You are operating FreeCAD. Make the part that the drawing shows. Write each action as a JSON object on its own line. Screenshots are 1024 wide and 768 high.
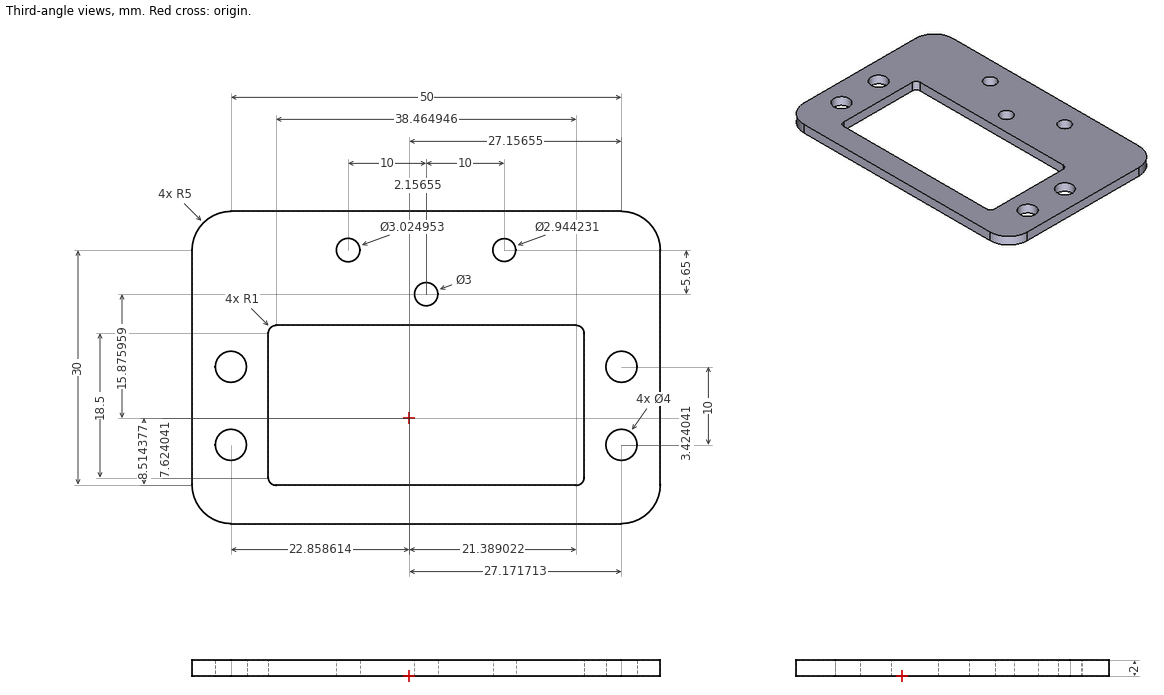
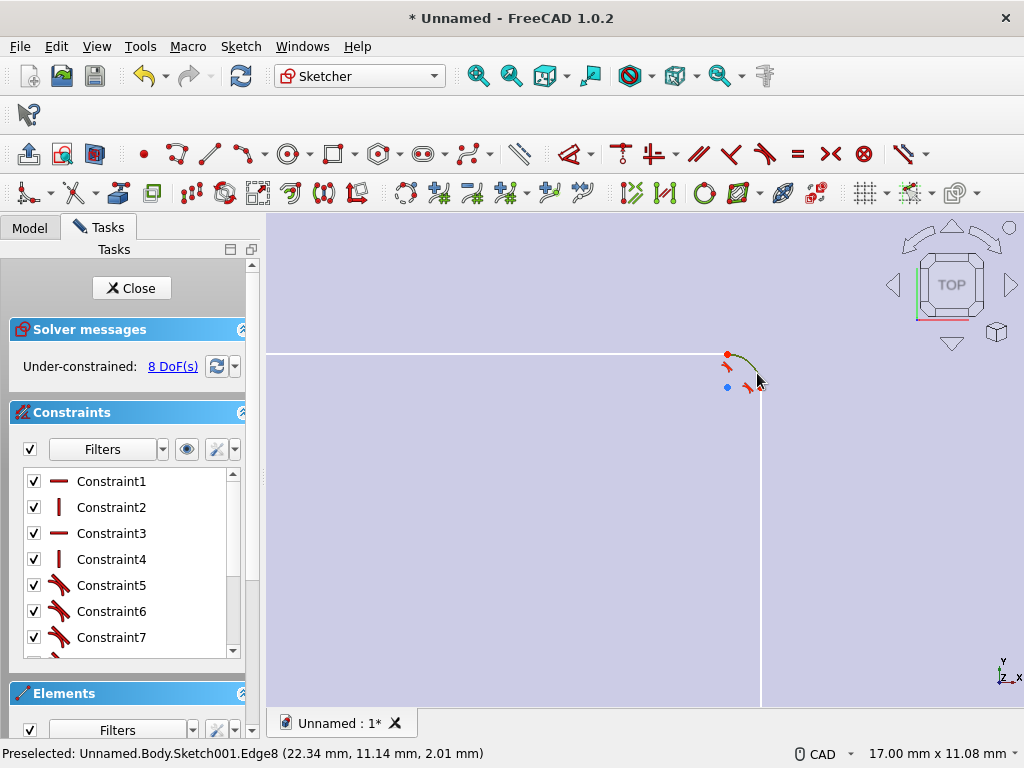
{"action": "left_click", "coordinate": [798, 154]}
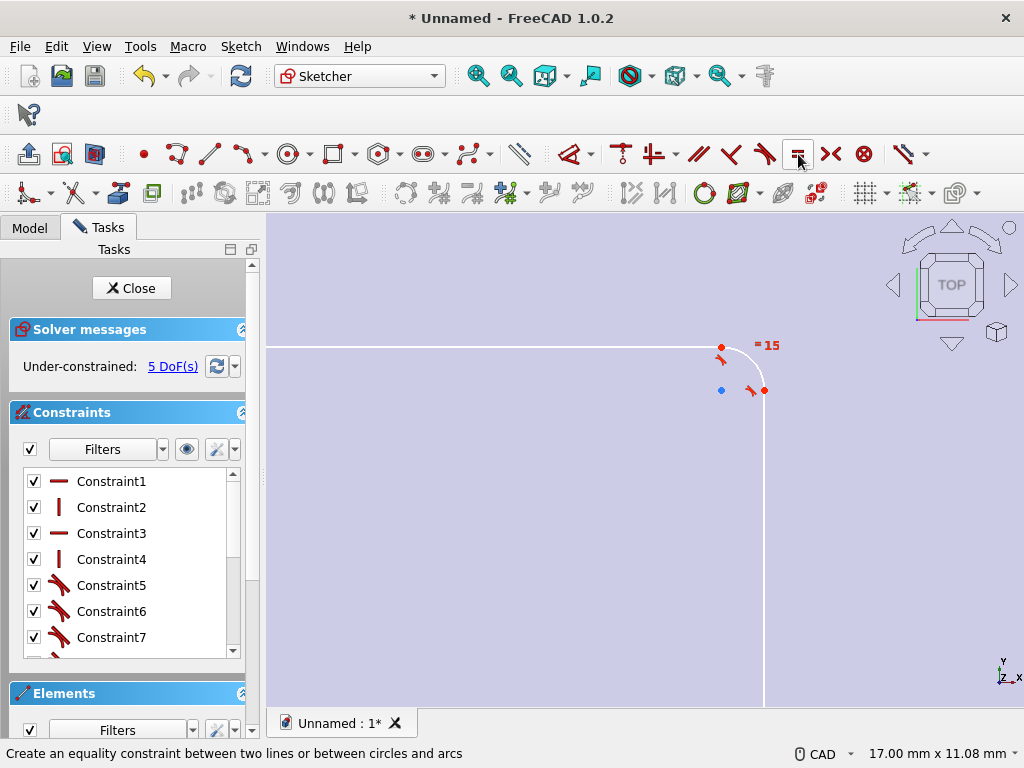
{"action": "left_click", "coordinate": [568, 154]}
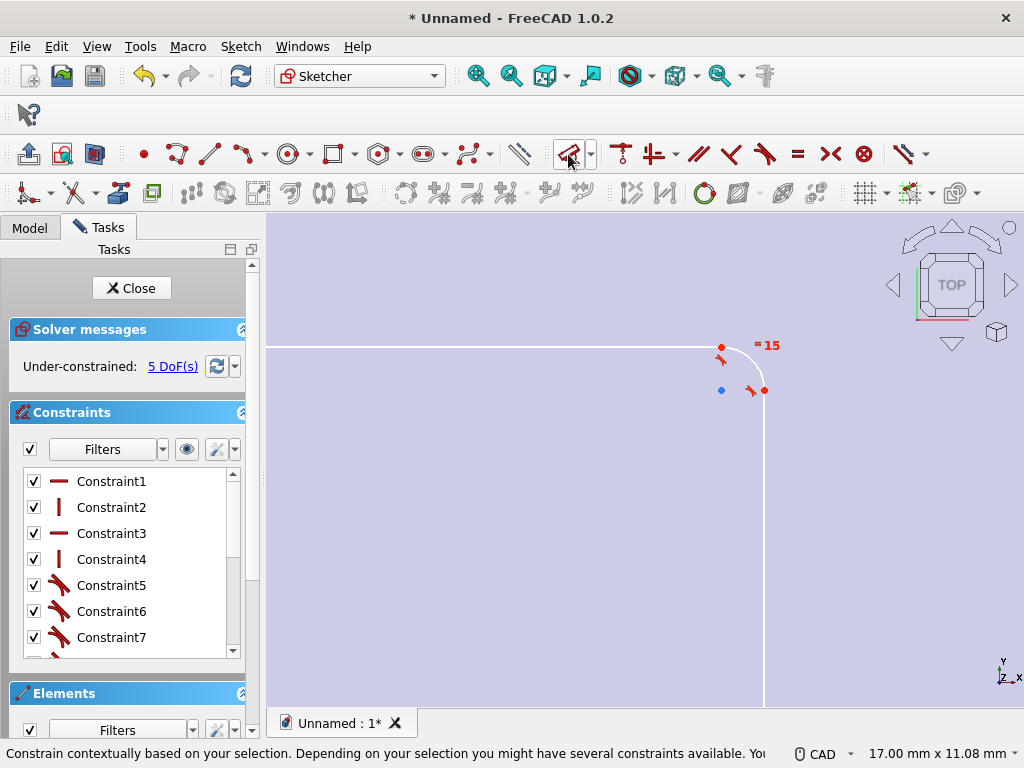
{"action": "scroll", "coordinate": [758, 374], "scroll_direction": "down", "scroll_amount": 8}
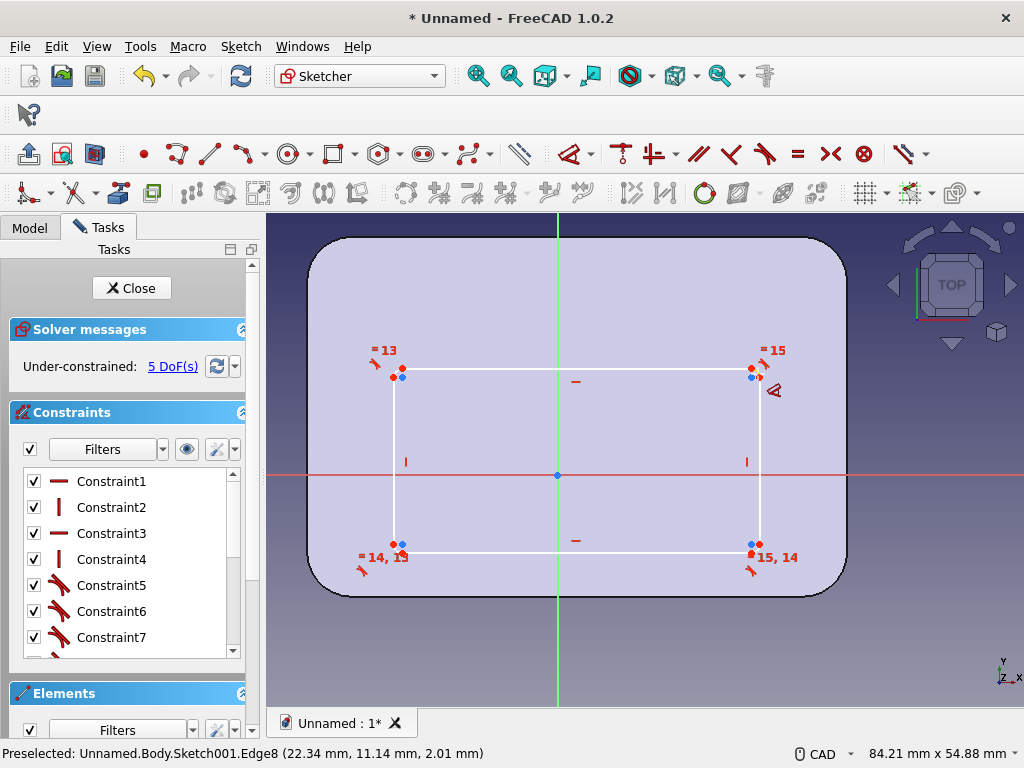
{"action": "scroll", "coordinate": [399, 370], "scroll_direction": "up", "scroll_amount": 8}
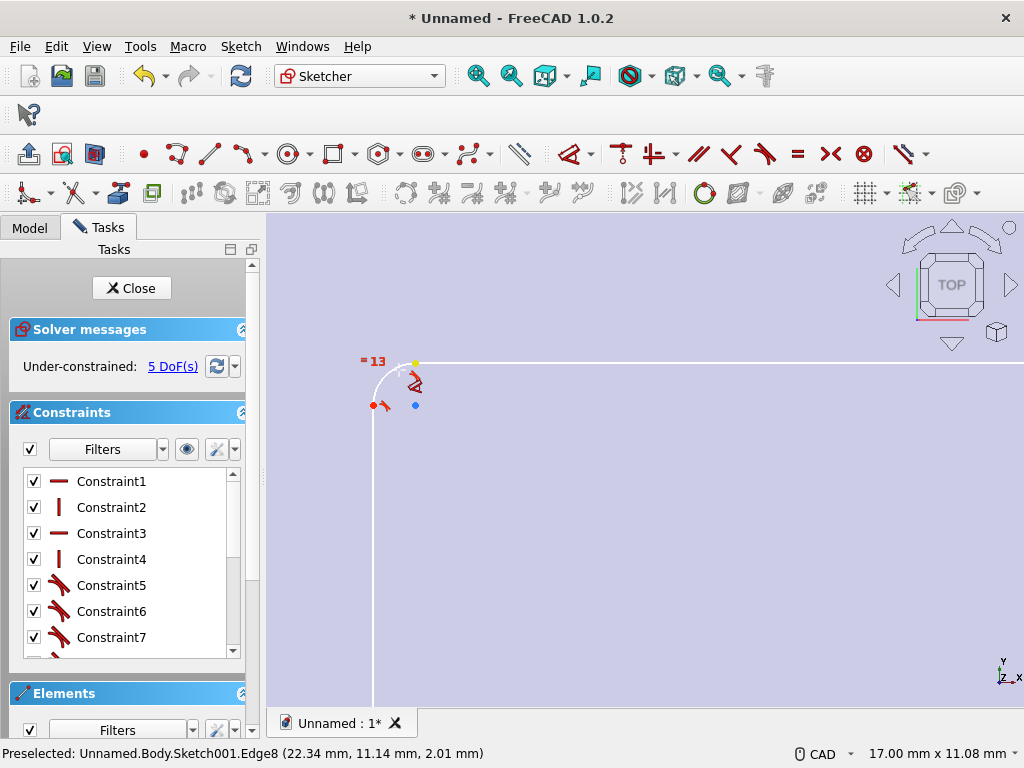
{"action": "left_click", "coordinate": [396, 368]}
{"action": "left_click", "coordinate": [381, 340]}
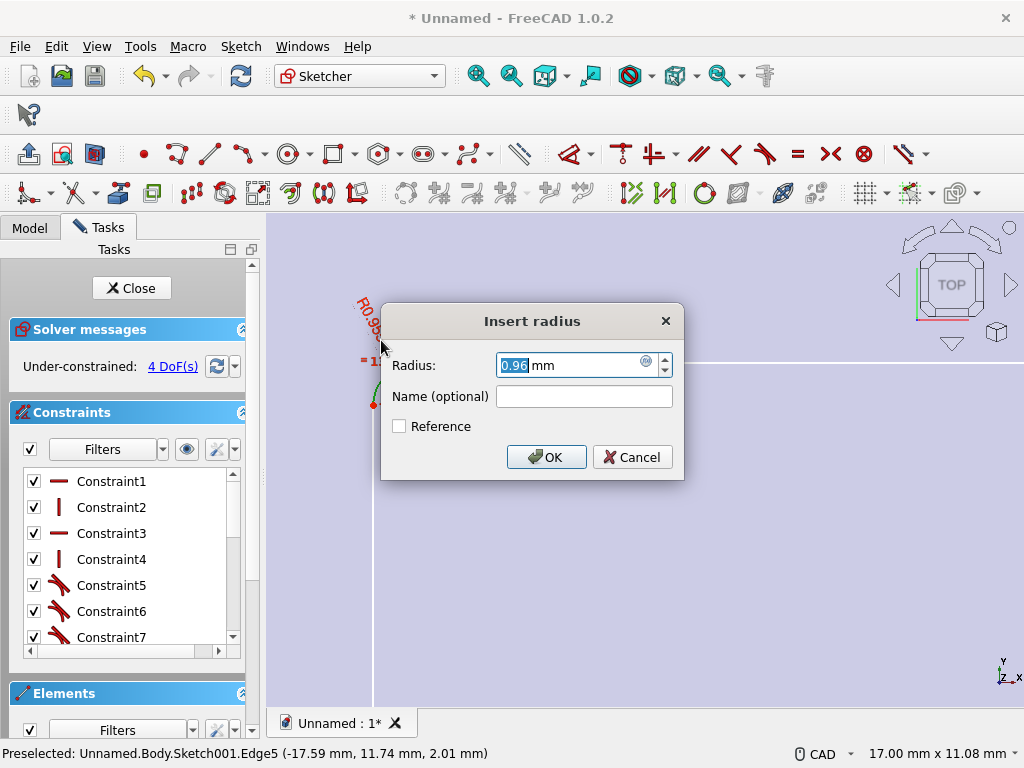
{"action": "type", "text": "1"}
{"action": "key", "text": "Return"}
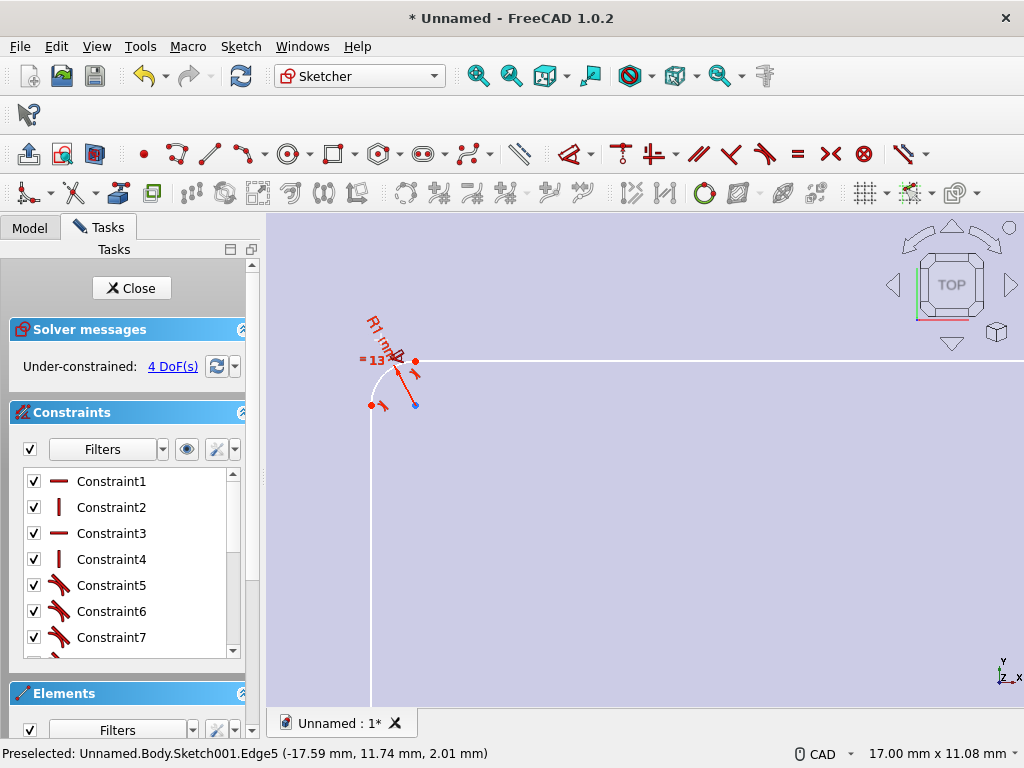
{"action": "scroll", "coordinate": [398, 370], "scroll_direction": "down", "scroll_amount": 8}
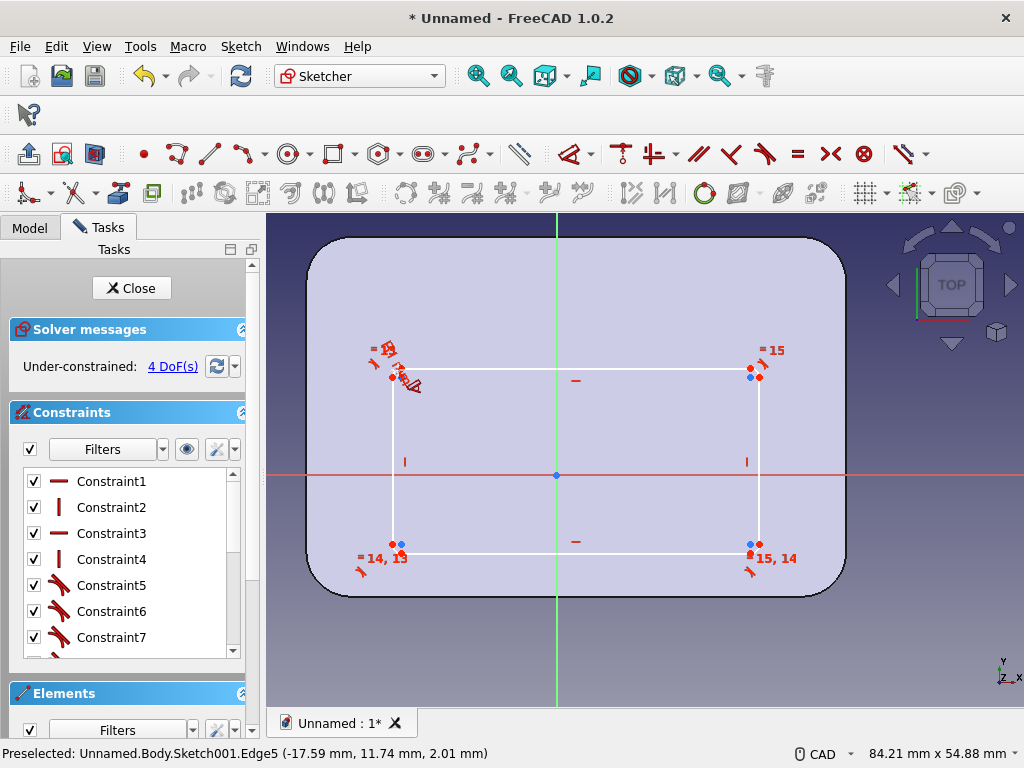
{"action": "left_click", "coordinate": [393, 428]}
{"action": "left_click", "coordinate": [359, 461]}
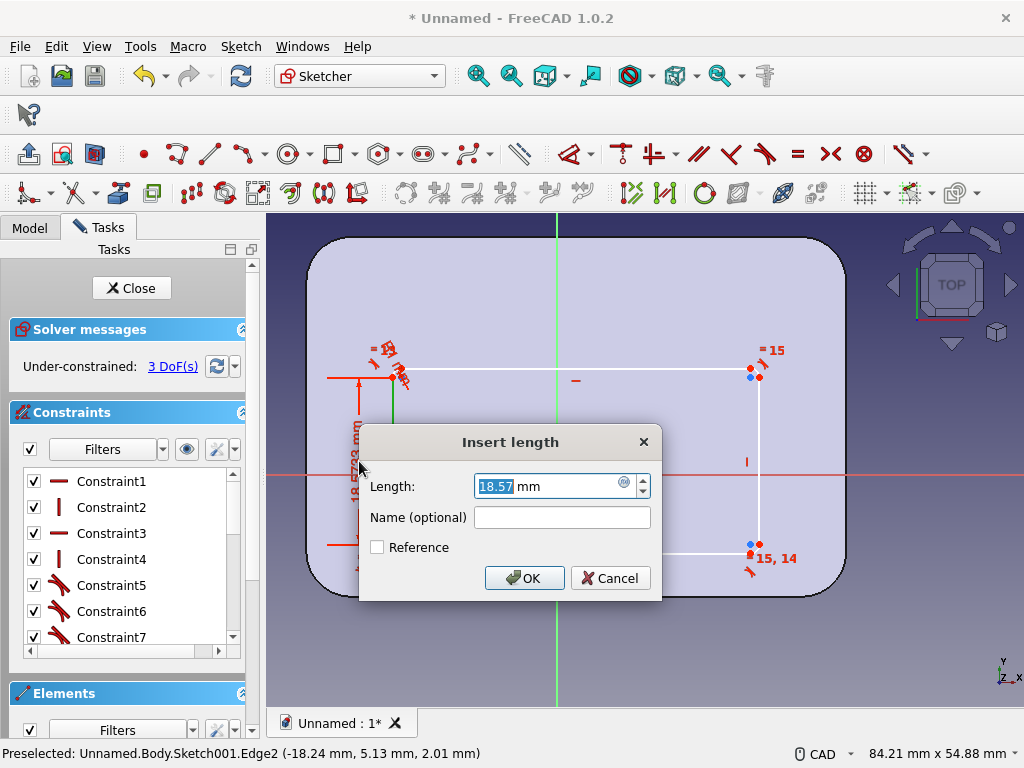
{"action": "type", "text": "18.5"}
{"action": "key", "text": "Return"}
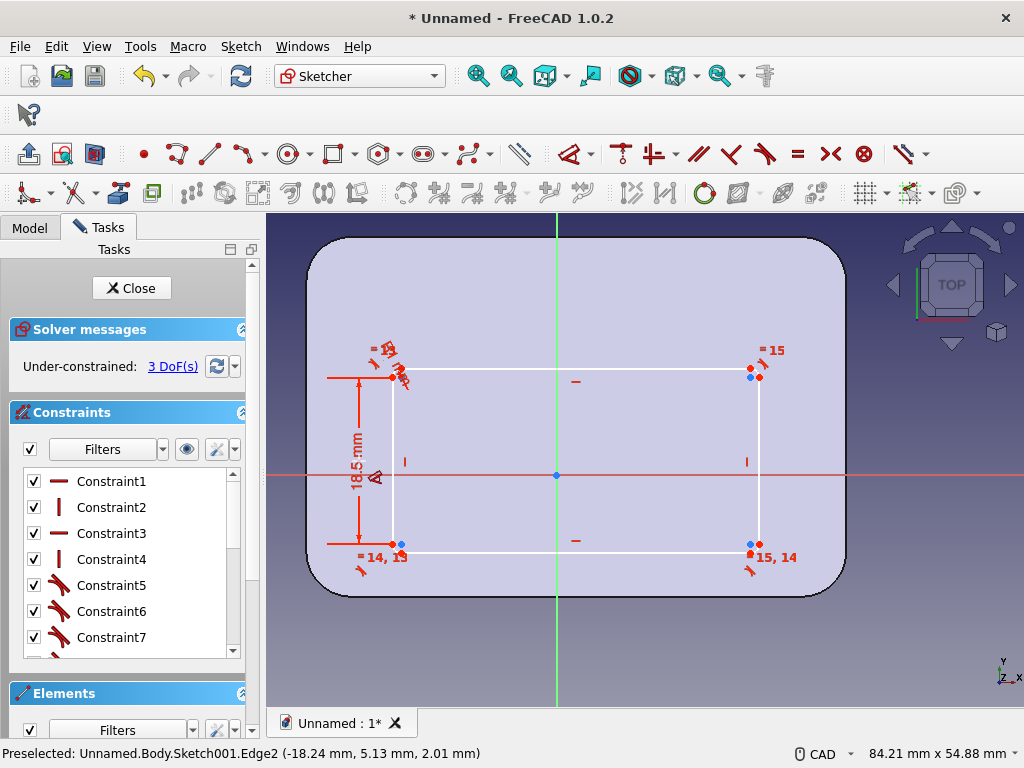
{"action": "left_click", "coordinate": [646, 369]}
{"action": "left_click", "coordinate": [576, 335]}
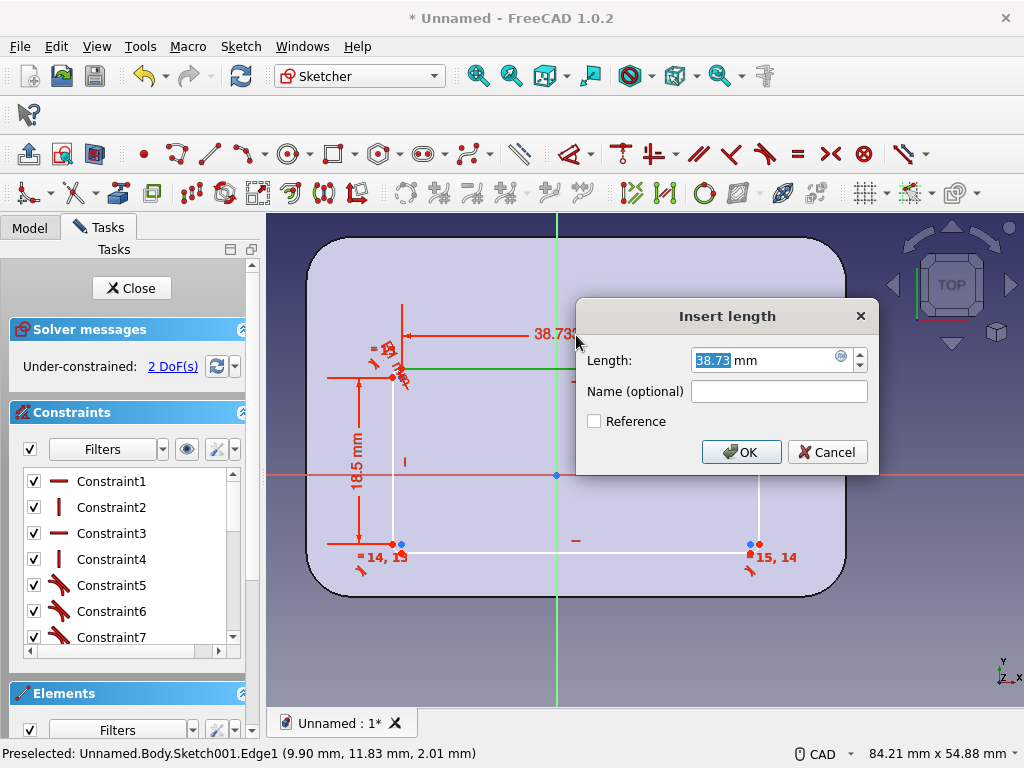
{"action": "type", "text": "38.464946"}
{"action": "key", "text": "Return"}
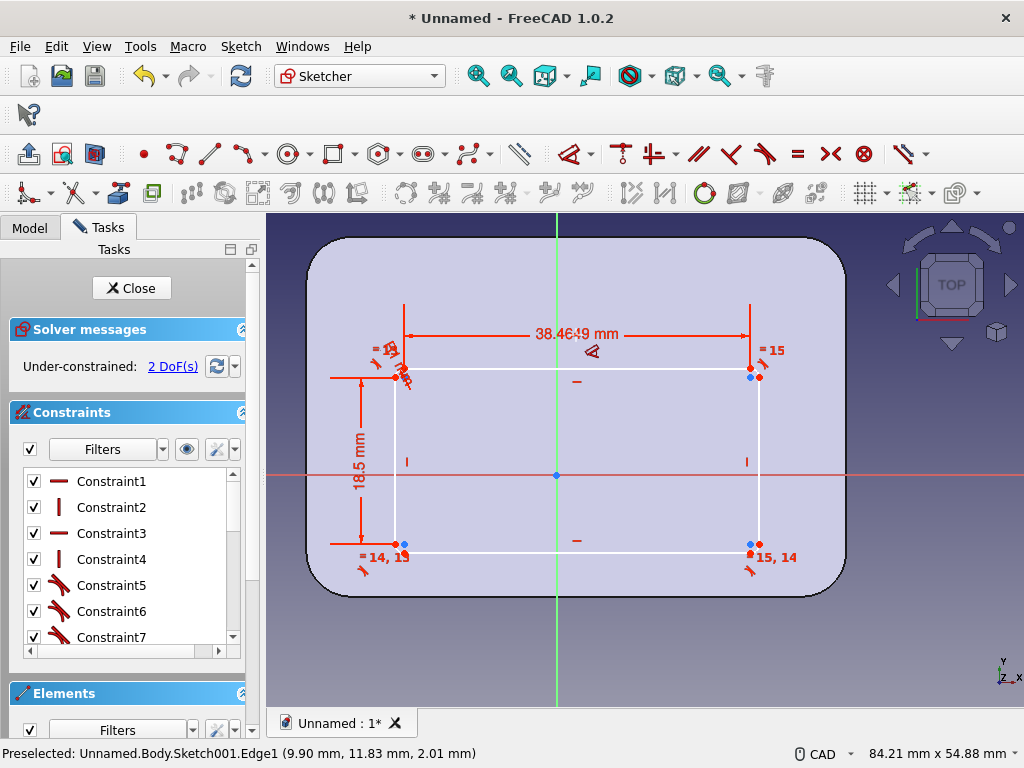
{"action": "scroll", "coordinate": [395, 544], "scroll_direction": "up", "scroll_amount": 2}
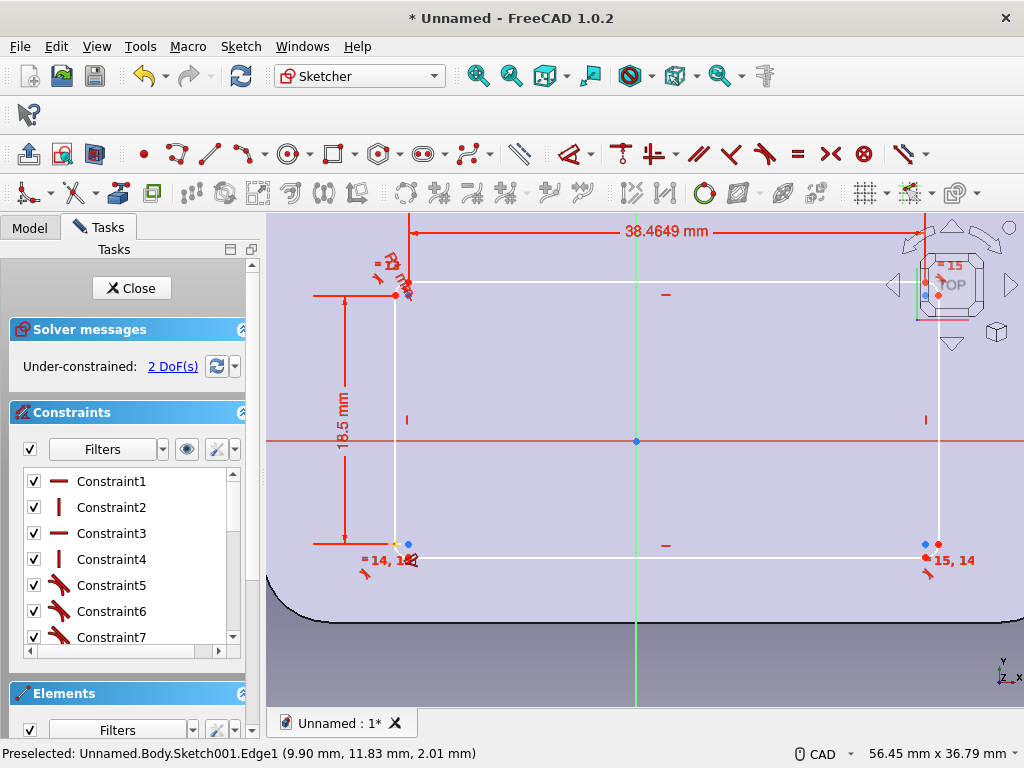
{"action": "left_click", "coordinate": [395, 544]}
{"action": "left_click", "coordinate": [361, 493]}